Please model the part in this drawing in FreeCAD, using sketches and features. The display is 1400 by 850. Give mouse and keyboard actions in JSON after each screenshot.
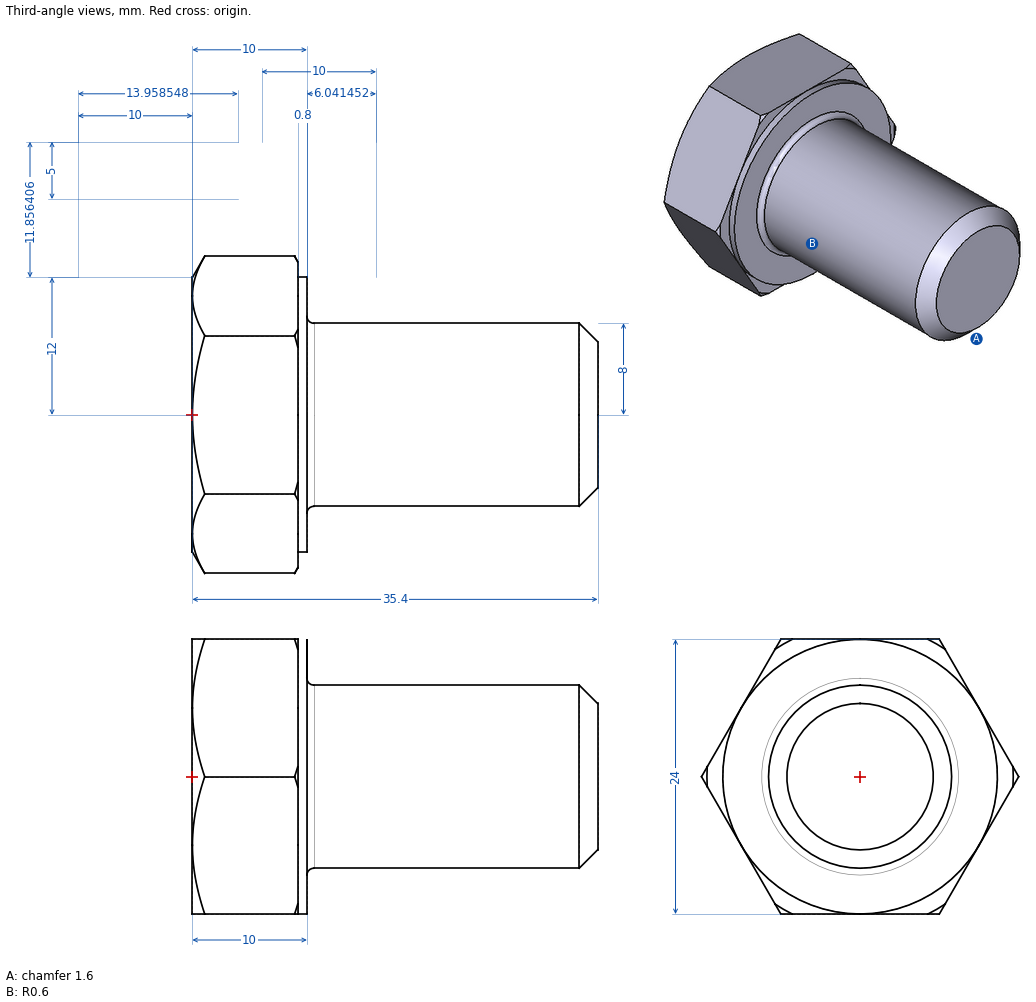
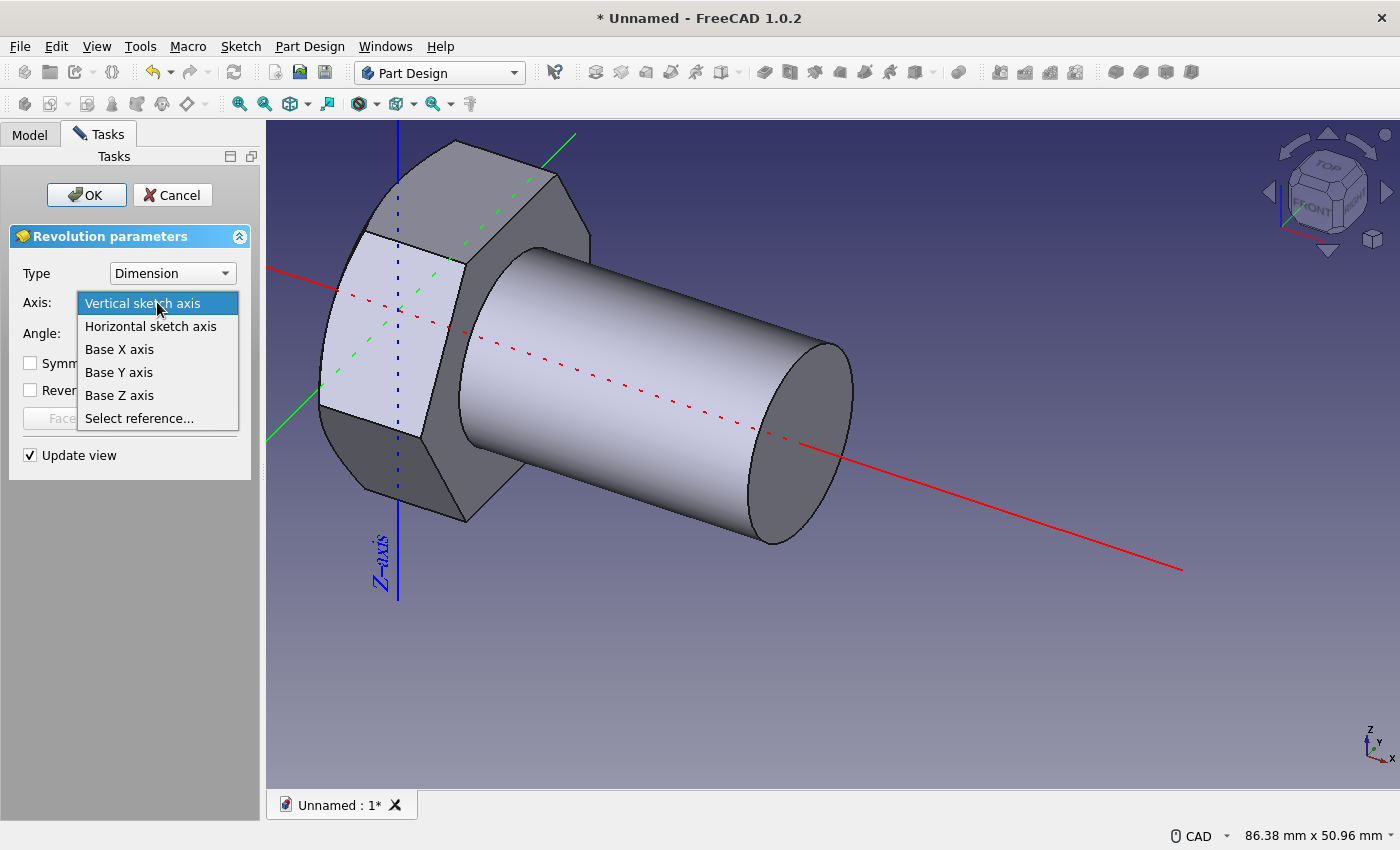
{"action": "left_click", "coordinate": [156, 326]}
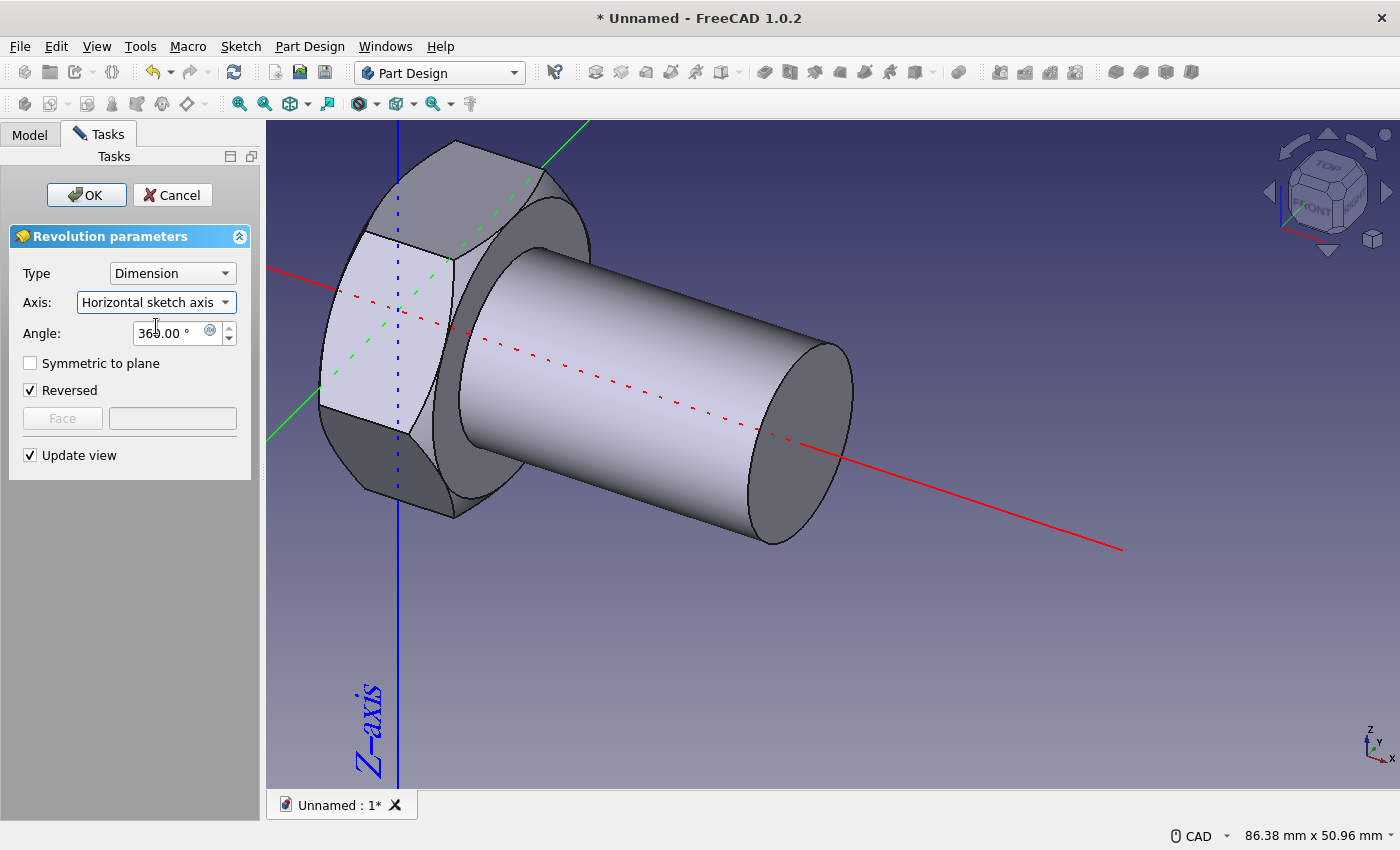
{"action": "left_click", "coordinate": [87, 195]}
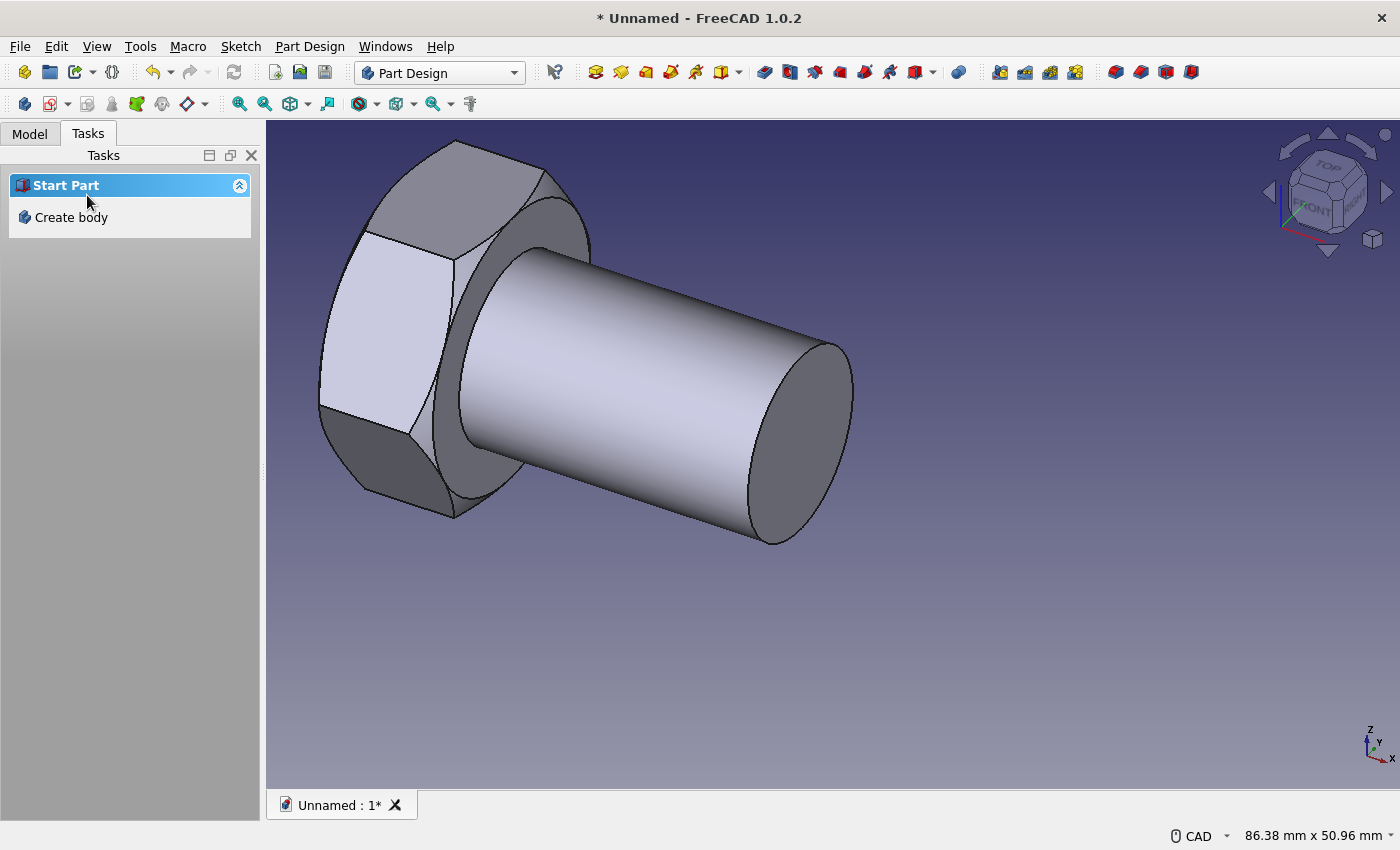
{"action": "key", "text": "v f"}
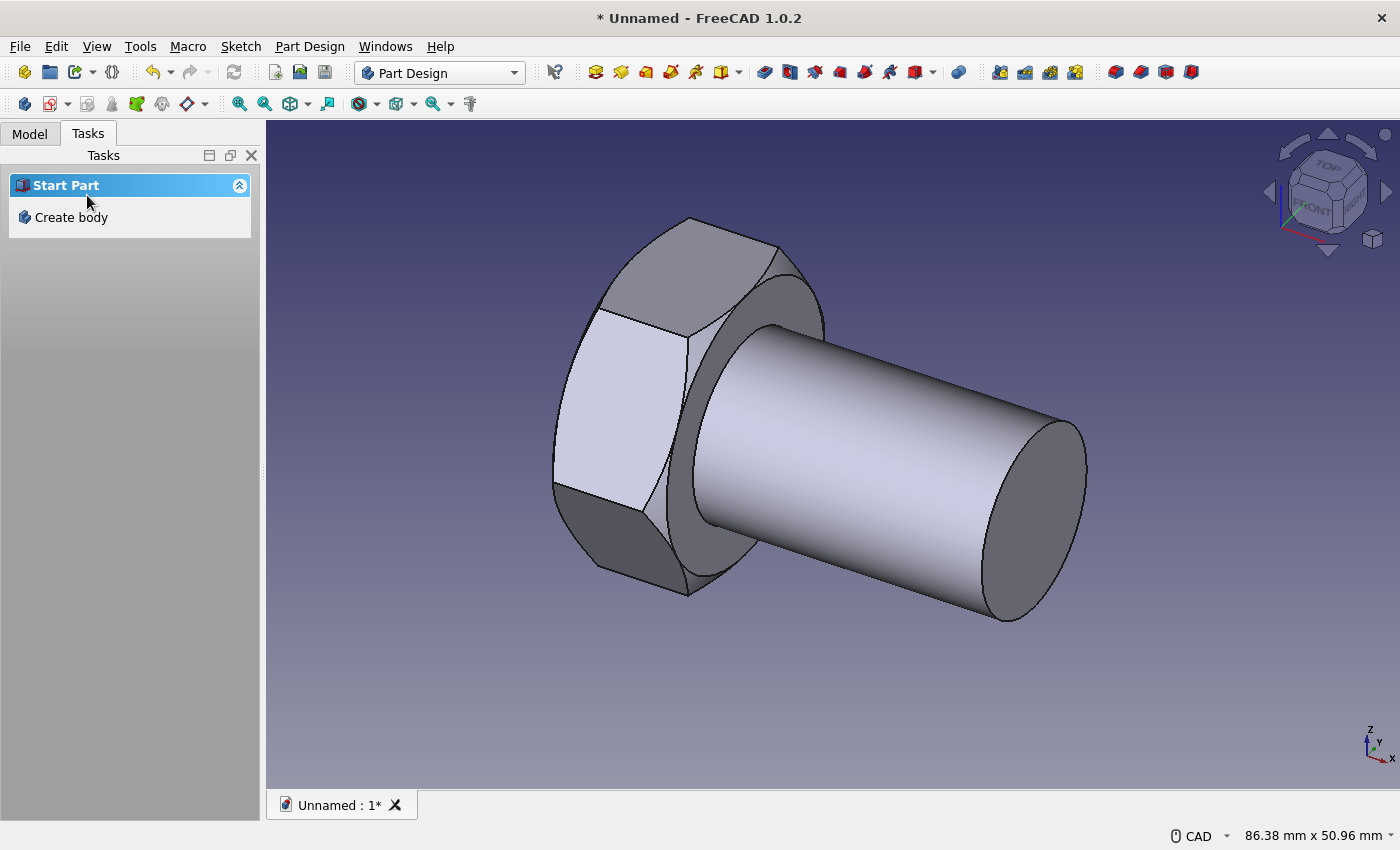
{"action": "left_click", "coordinate": [50, 104]}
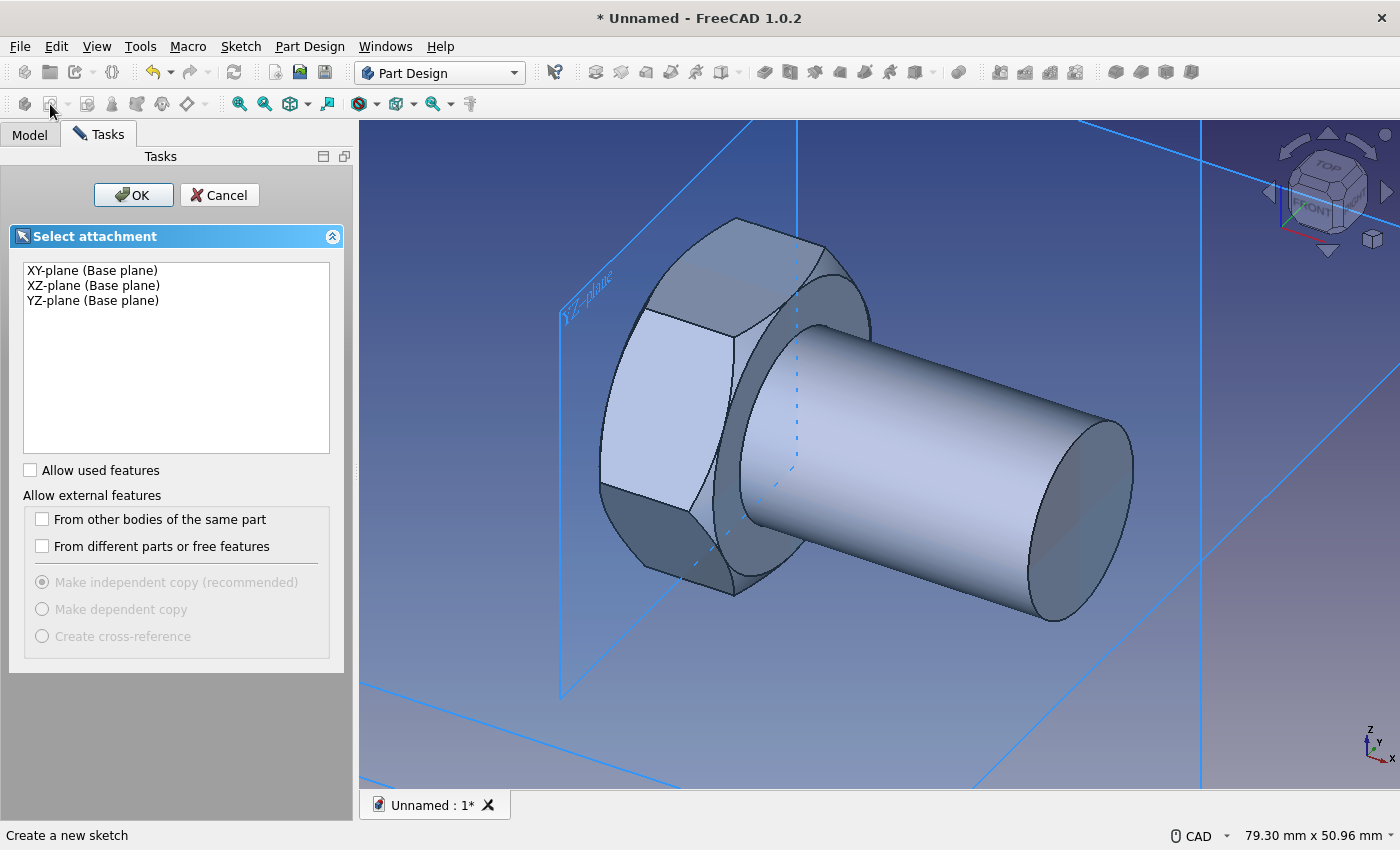
{"action": "left_click", "coordinate": [84, 270]}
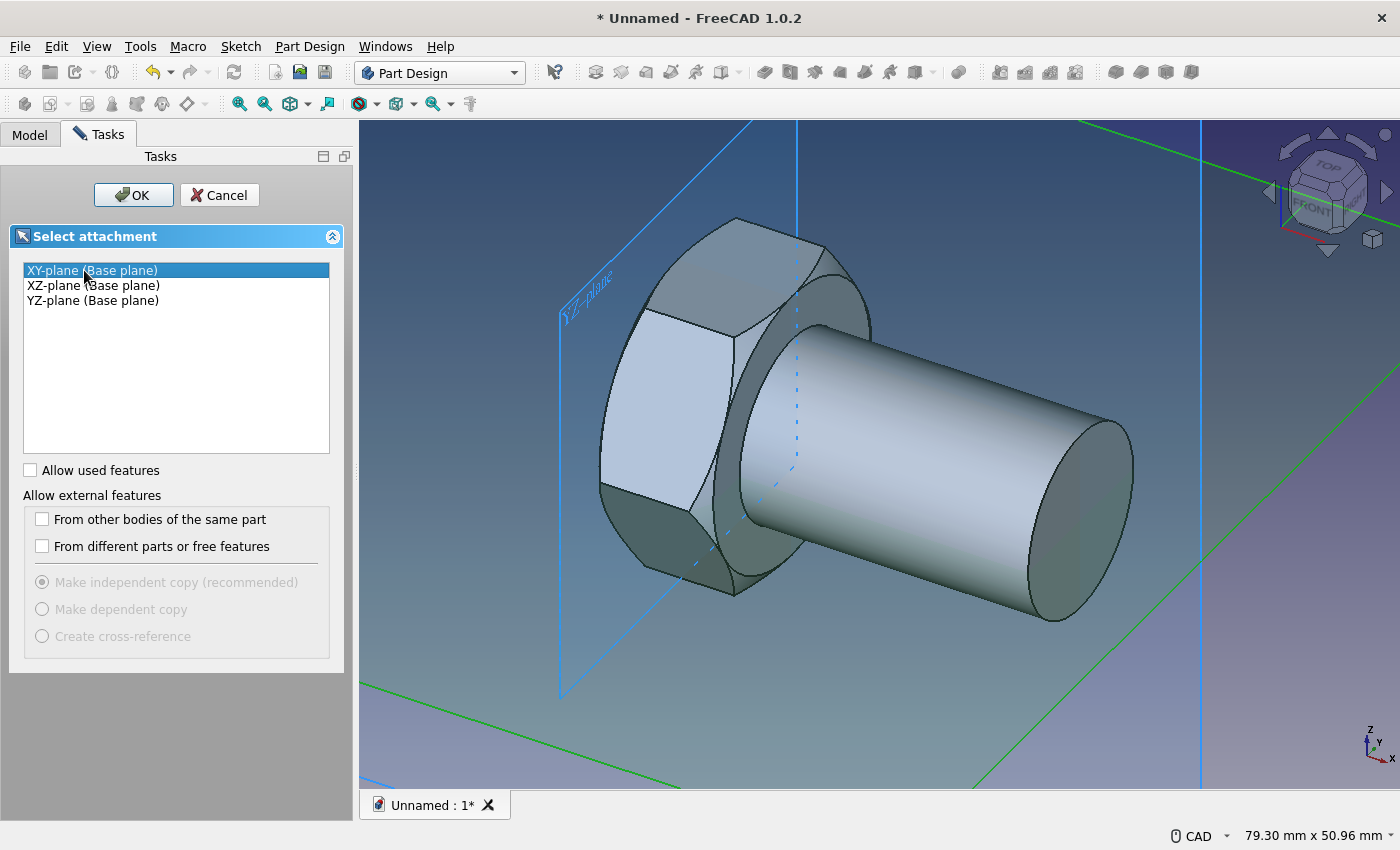
{"action": "left_click", "coordinate": [134, 195]}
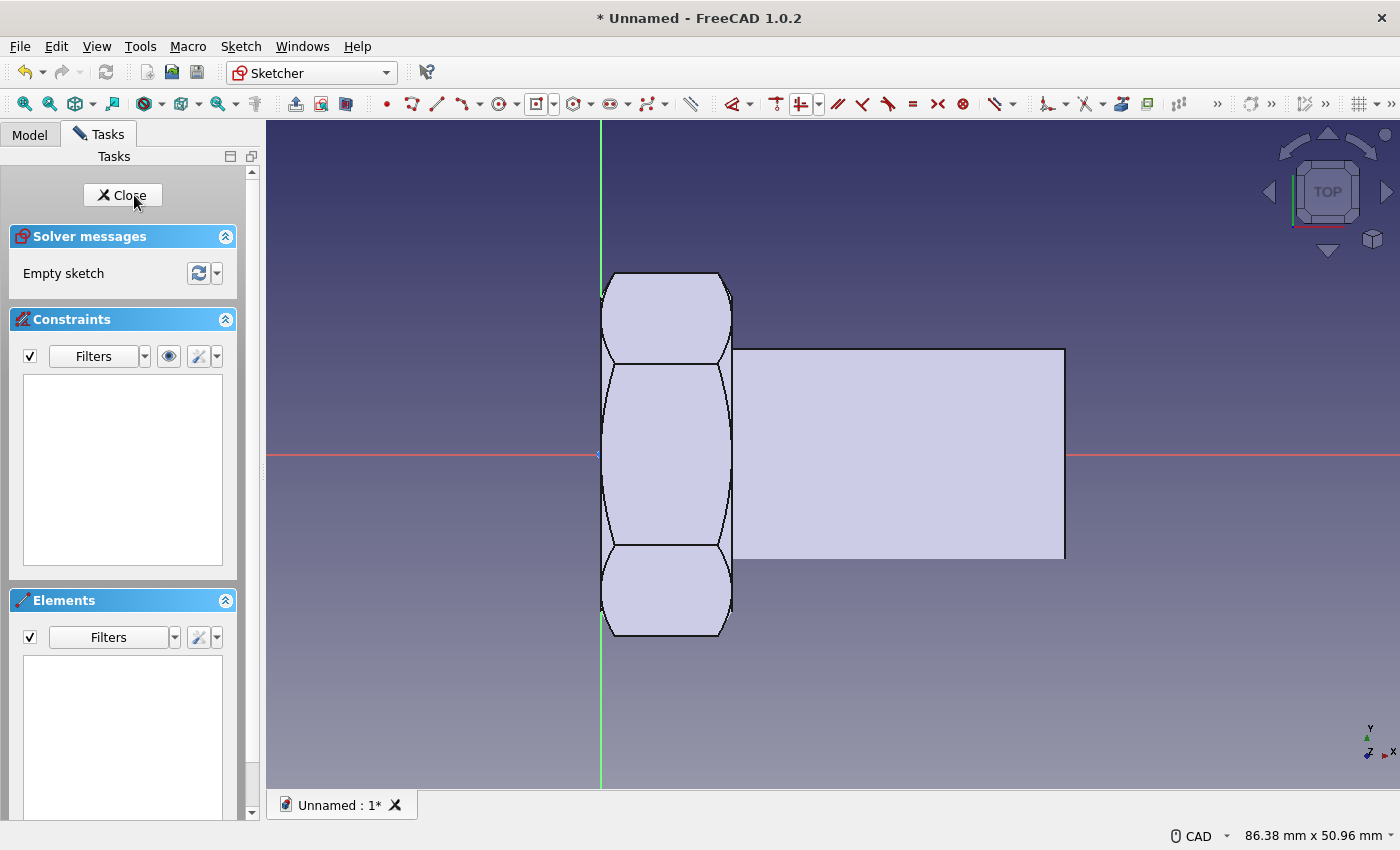
{"action": "key", "text": "q s"}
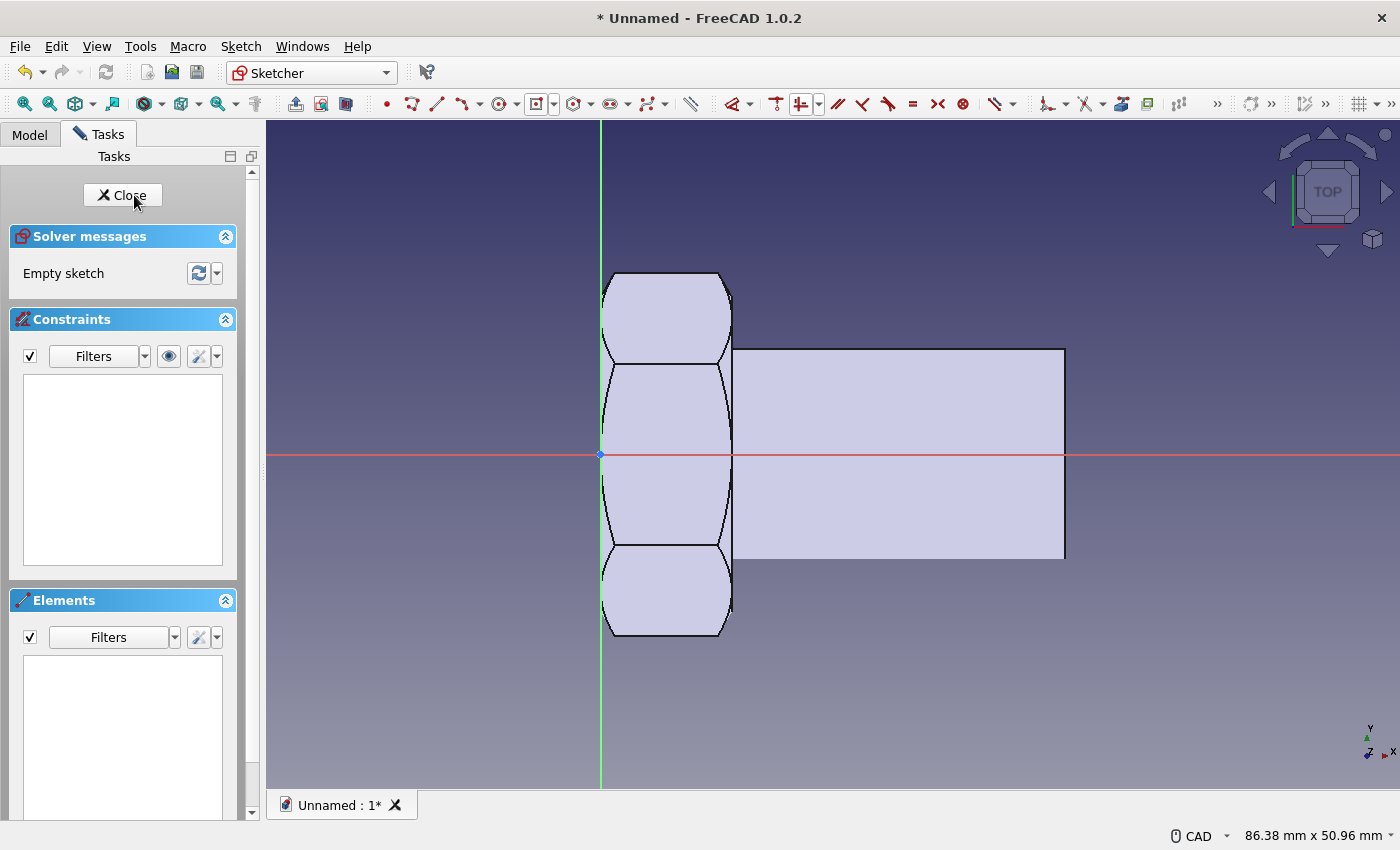
{"action": "scroll", "coordinate": [1208, 761], "scroll_direction": "down", "scroll_amount": 1}